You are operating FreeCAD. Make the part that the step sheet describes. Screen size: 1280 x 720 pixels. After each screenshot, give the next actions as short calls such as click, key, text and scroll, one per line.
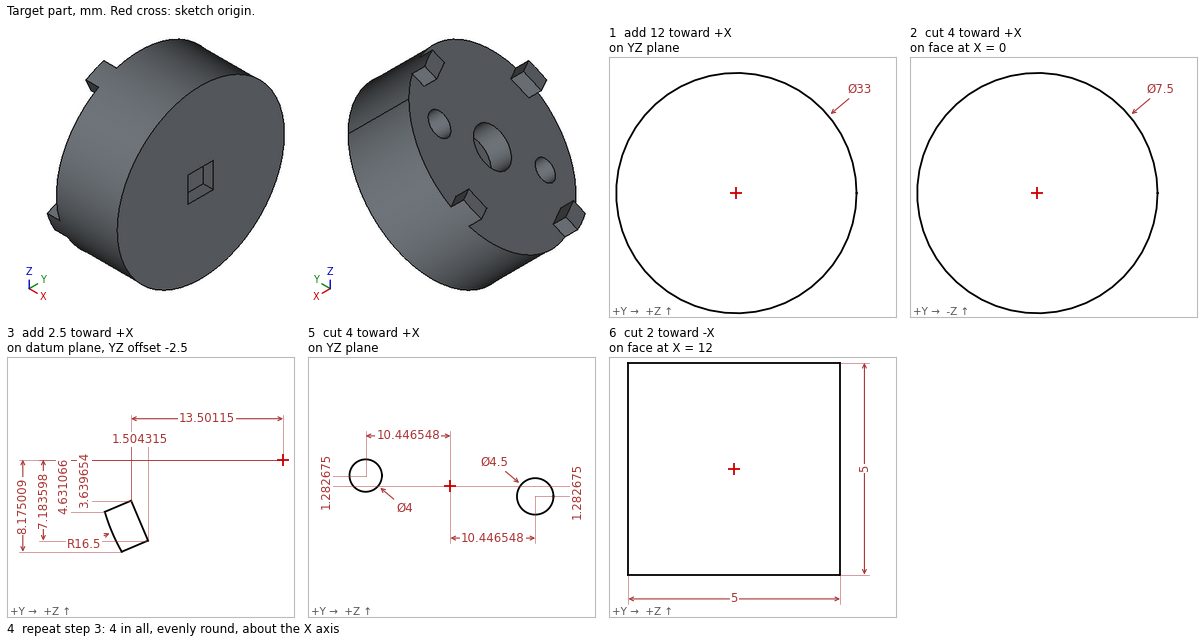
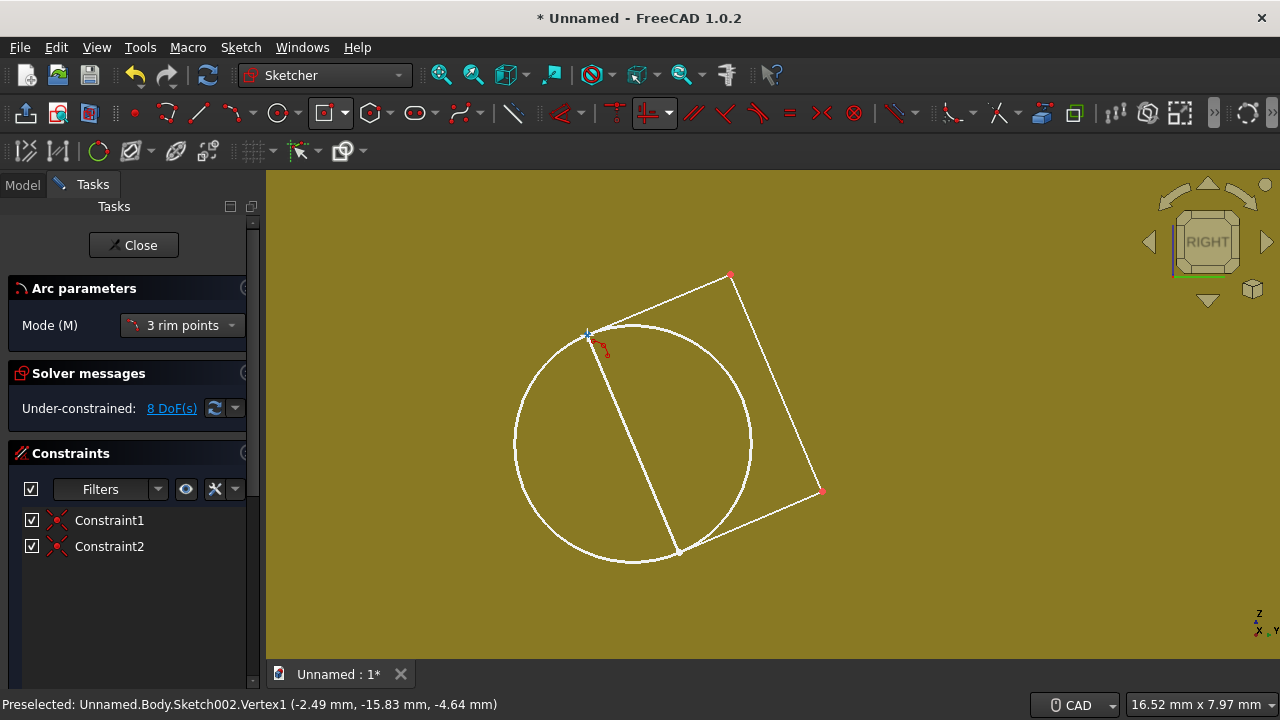
scroll(627, 446, up, 5)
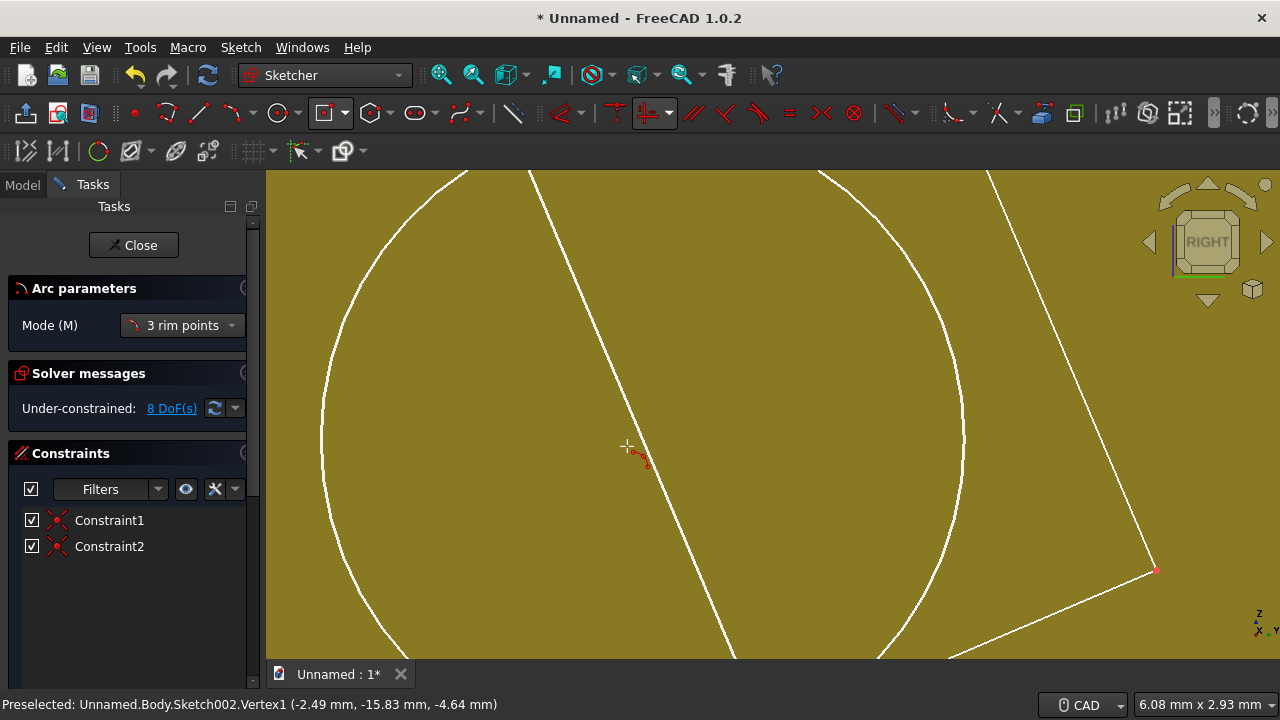
click(625, 445)
key(Escape)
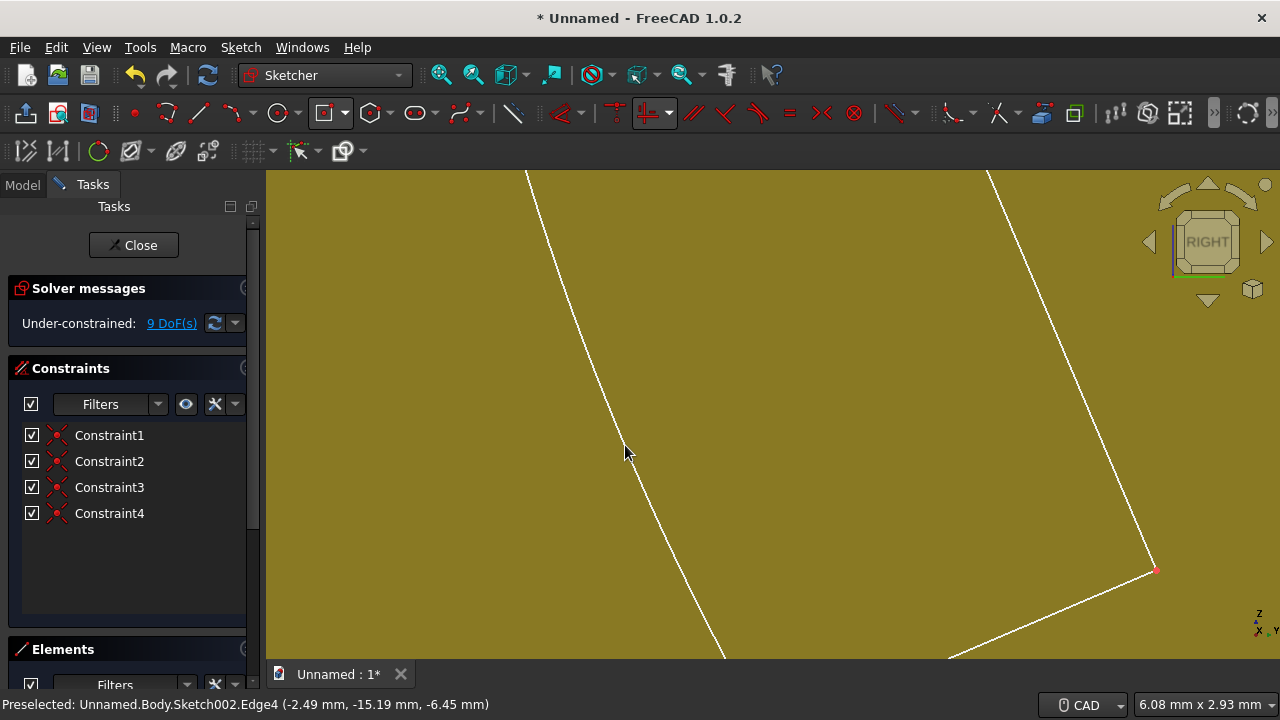
scroll(627, 449, down, 5)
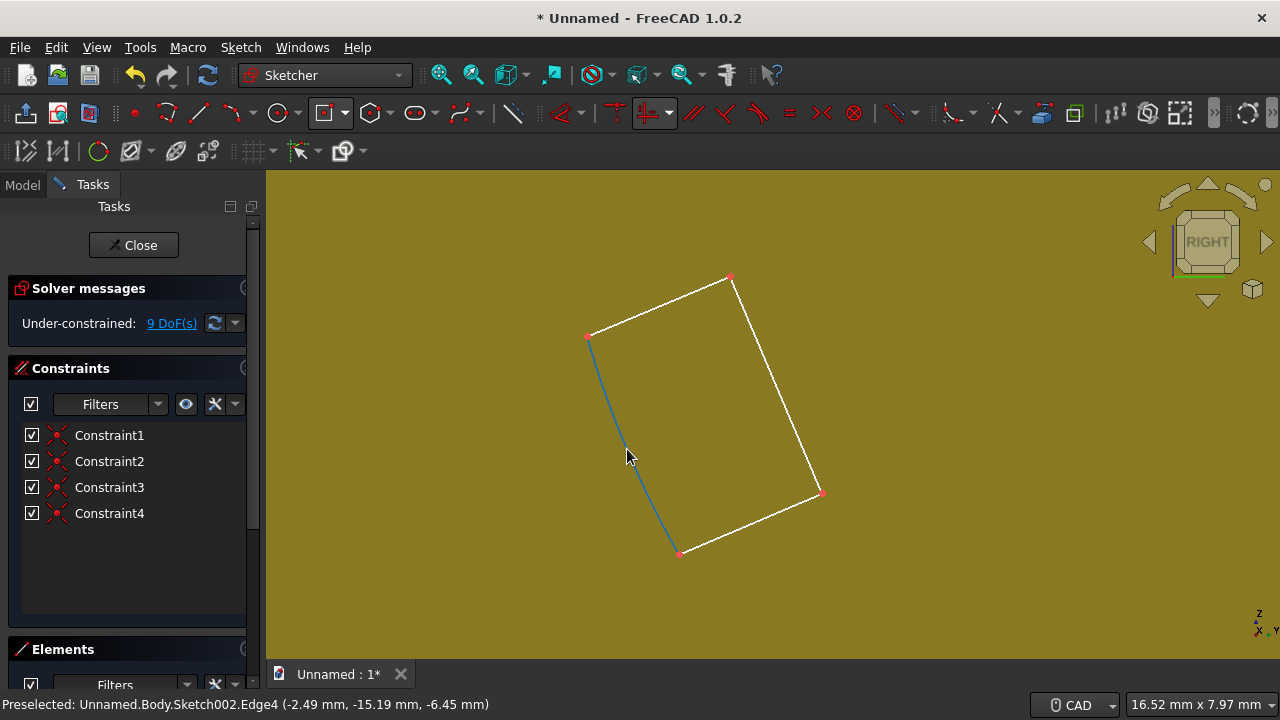
scroll(294, 550, down, 3)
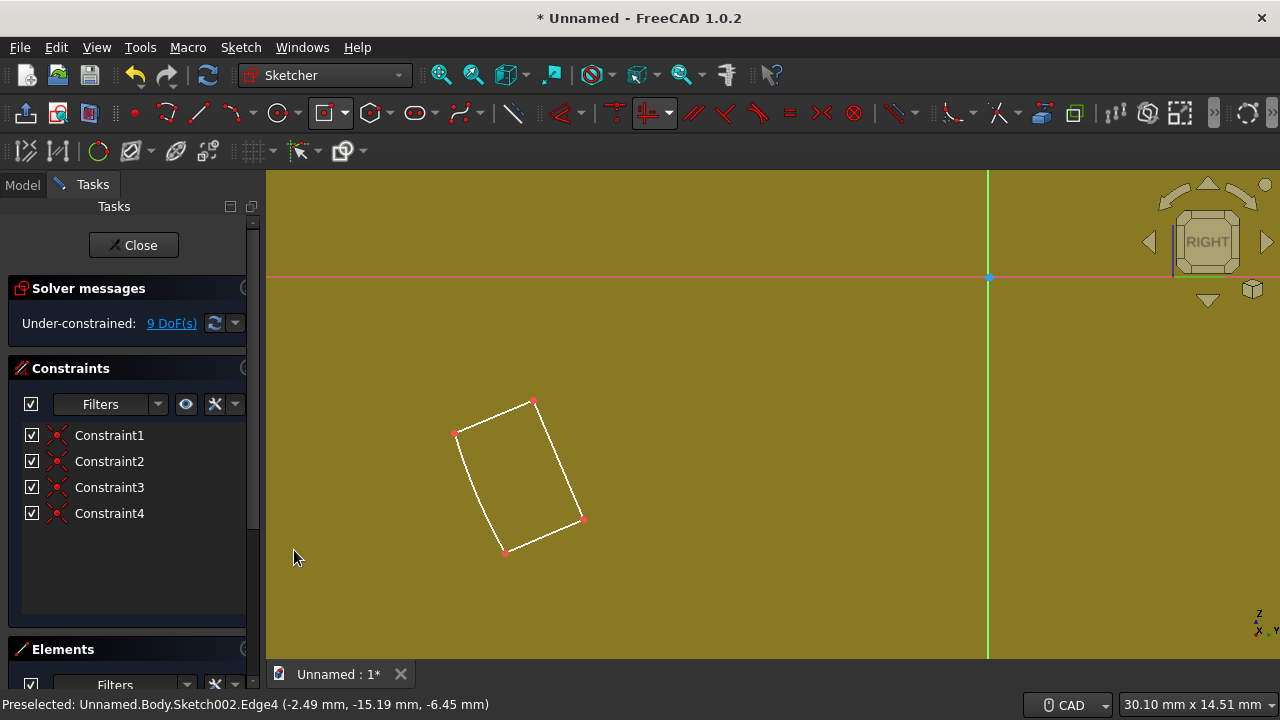
drag(978, 267, 1000, 288)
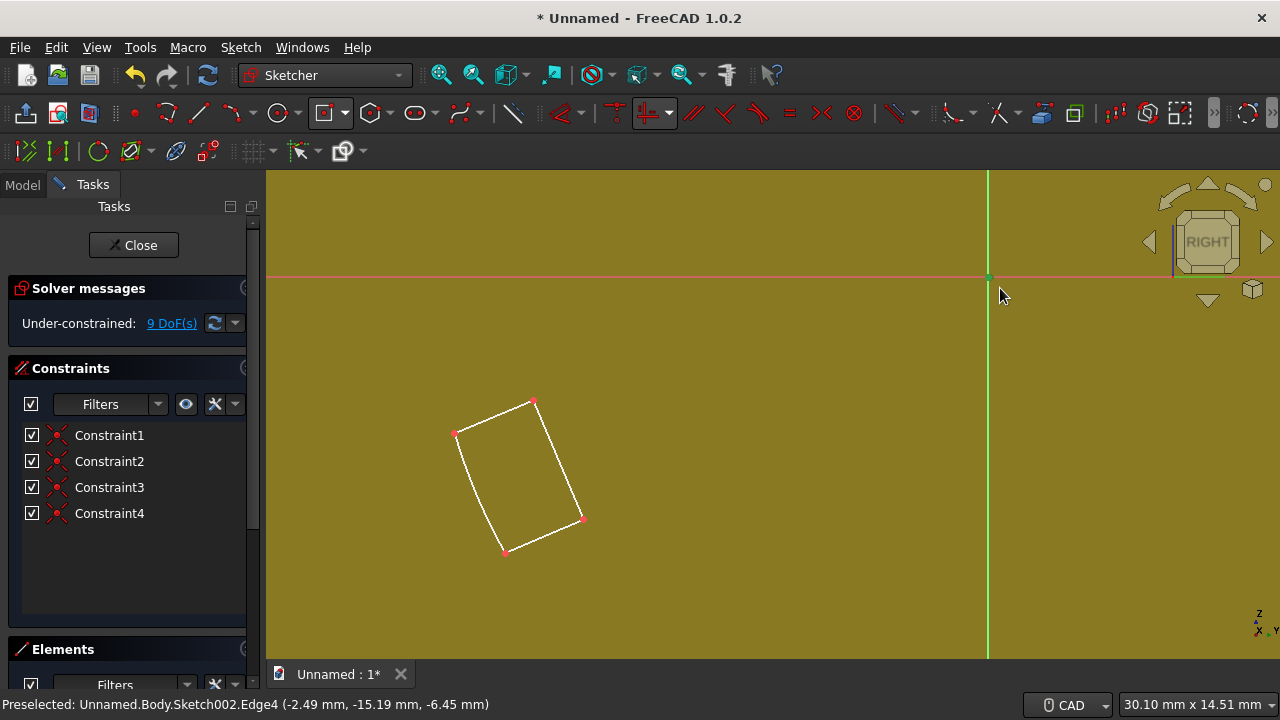
click(616, 114)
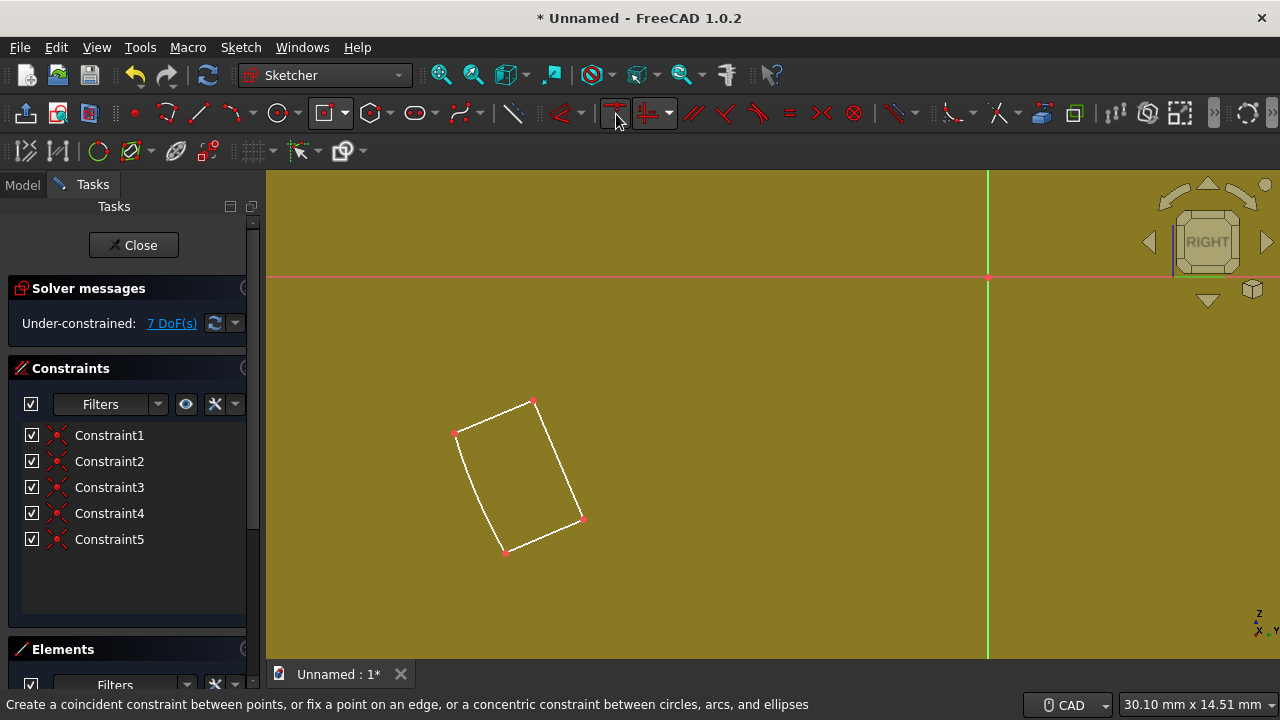
key(d)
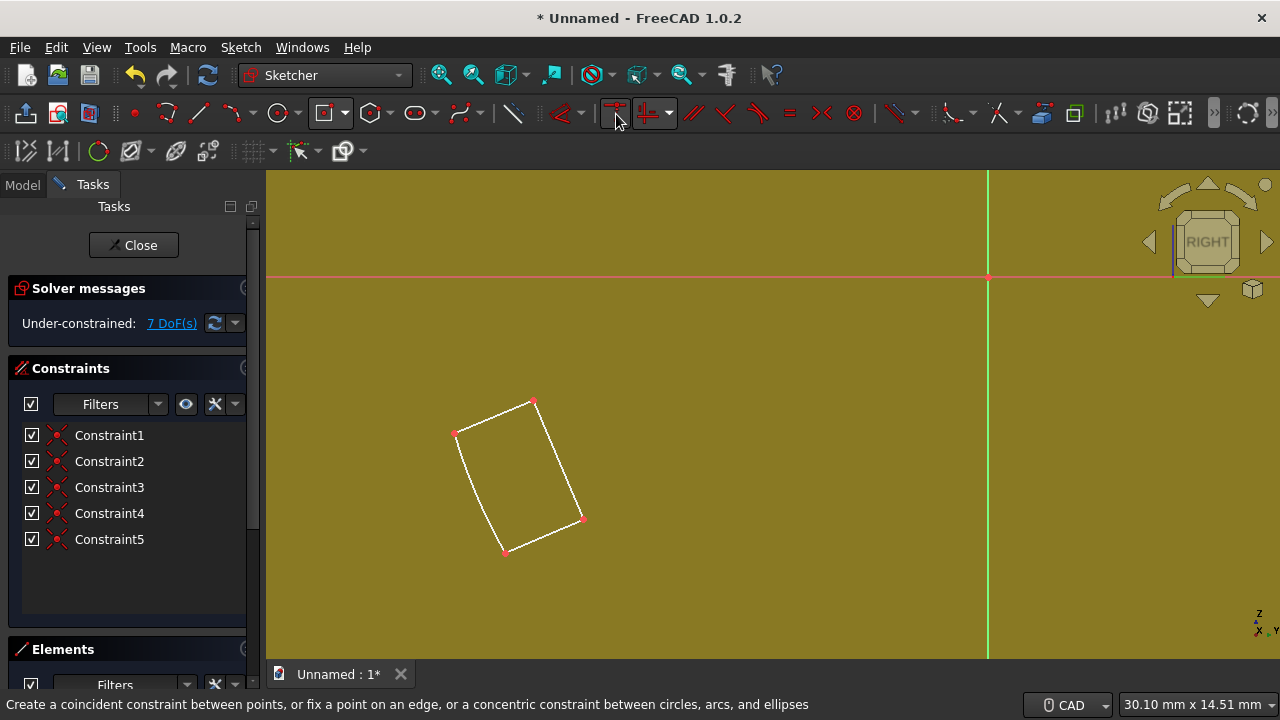
click(467, 470)
click(437, 481)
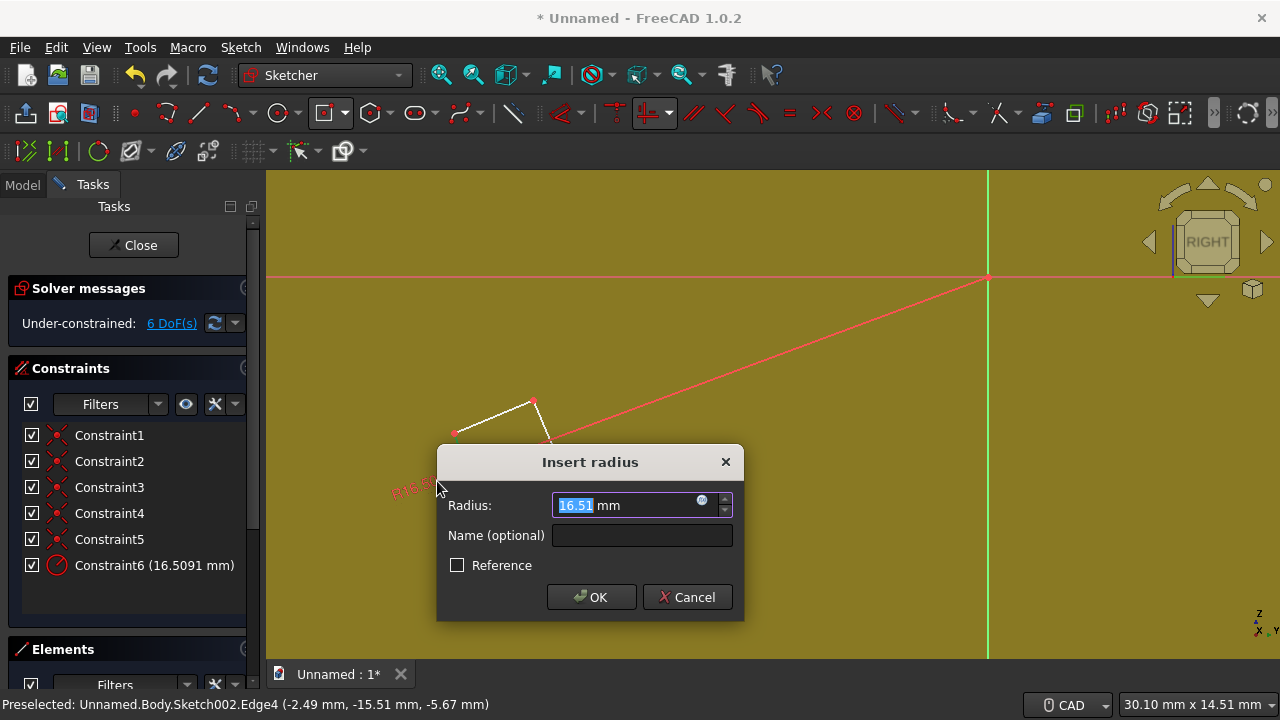
text(16.5)
key(Return)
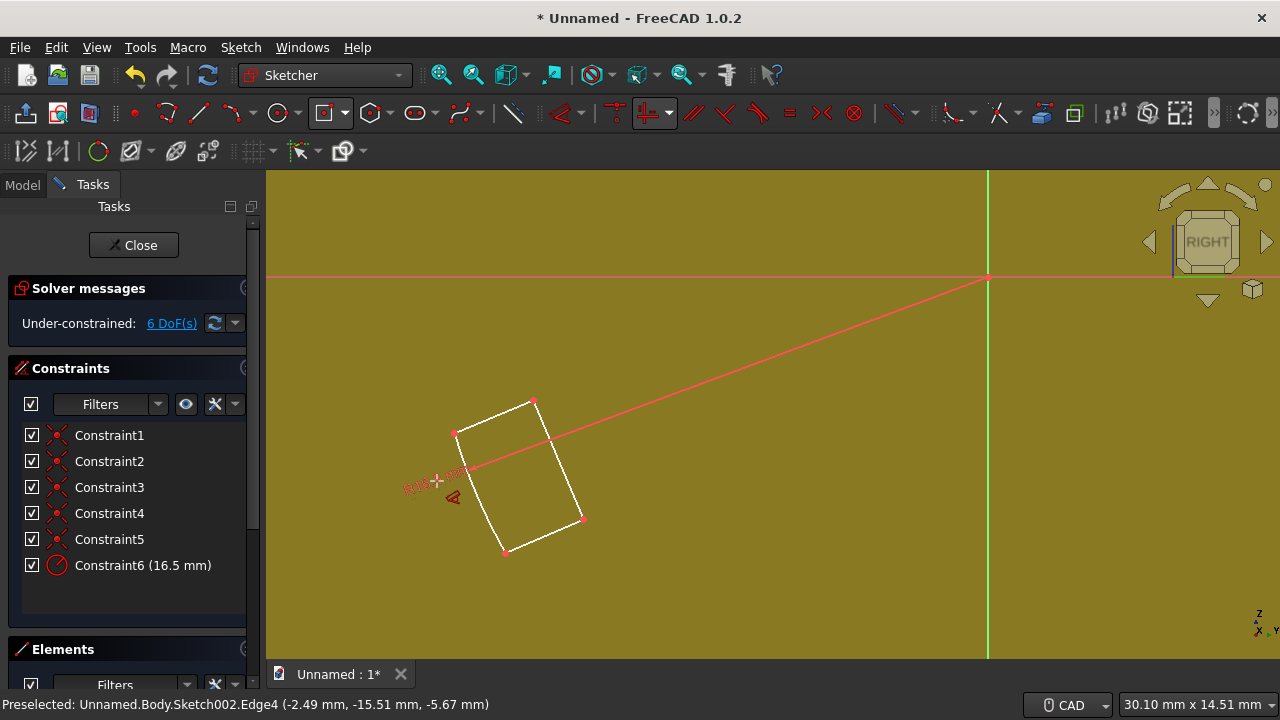
click(455, 433)
click(1022, 355)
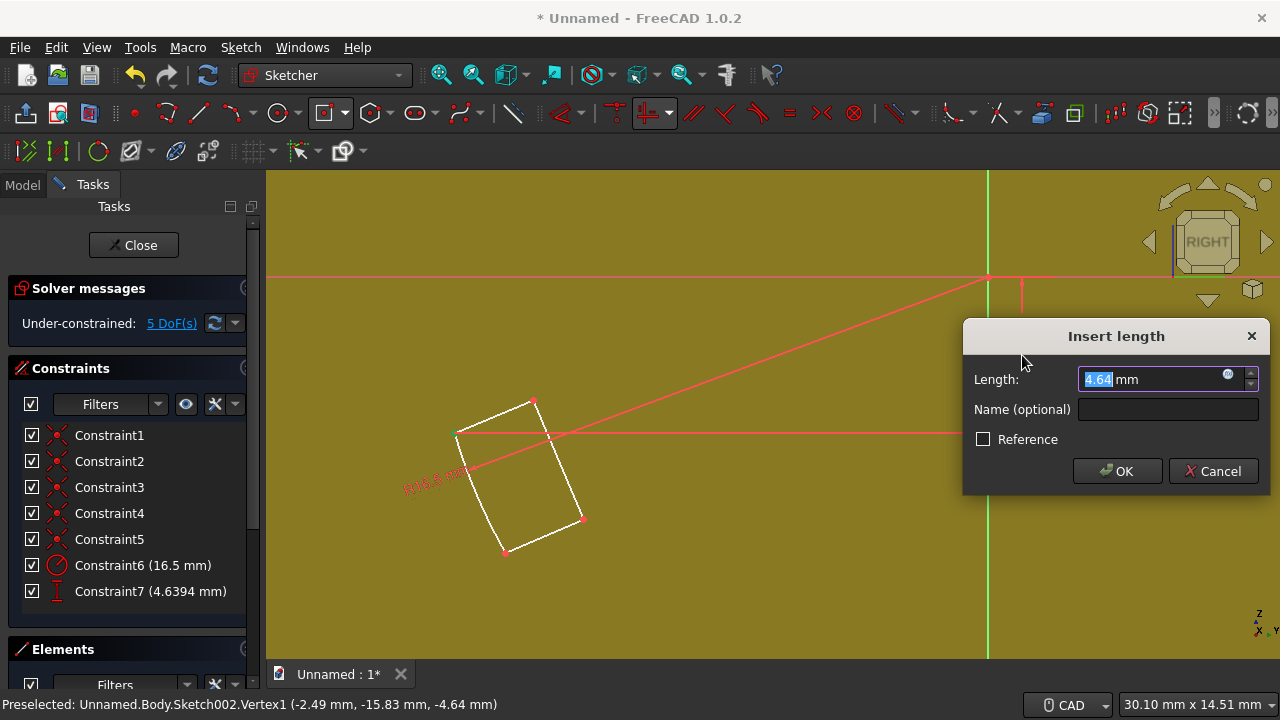
text(4.631066)
key(Return)